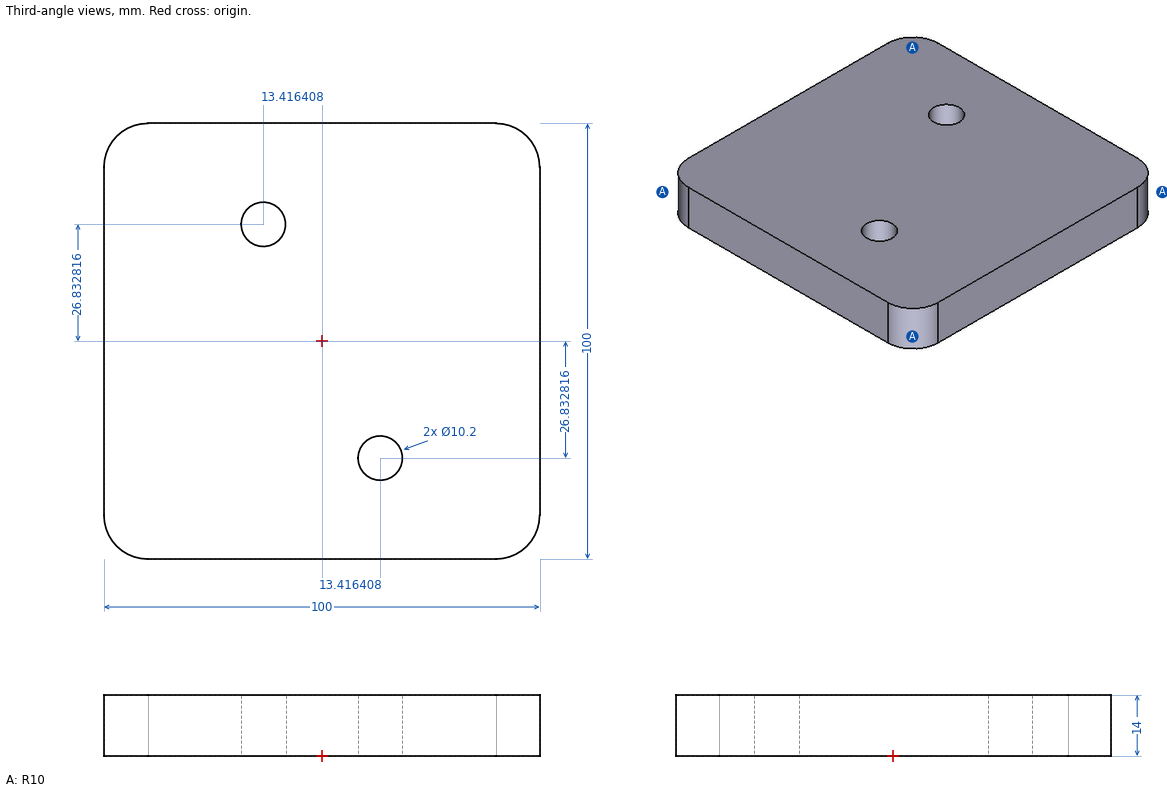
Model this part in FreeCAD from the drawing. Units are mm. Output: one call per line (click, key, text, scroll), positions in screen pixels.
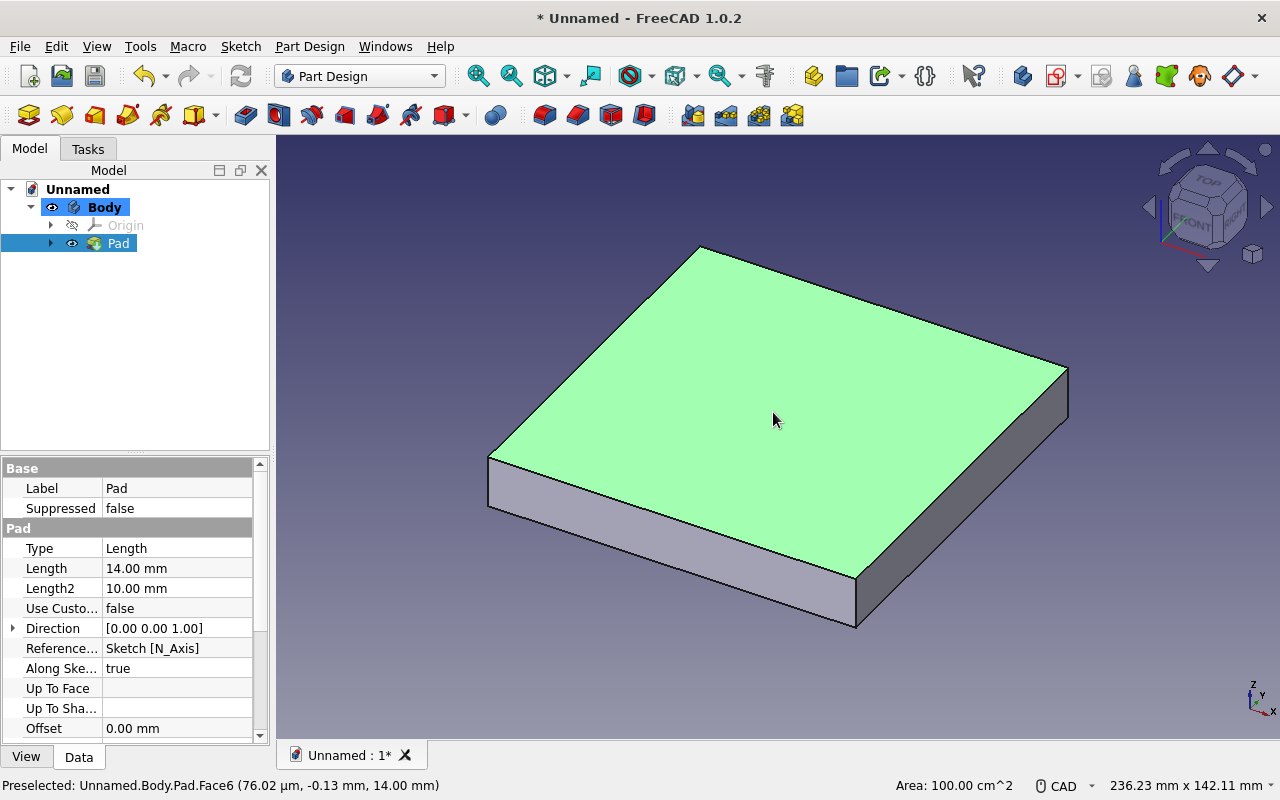
click(1056, 76)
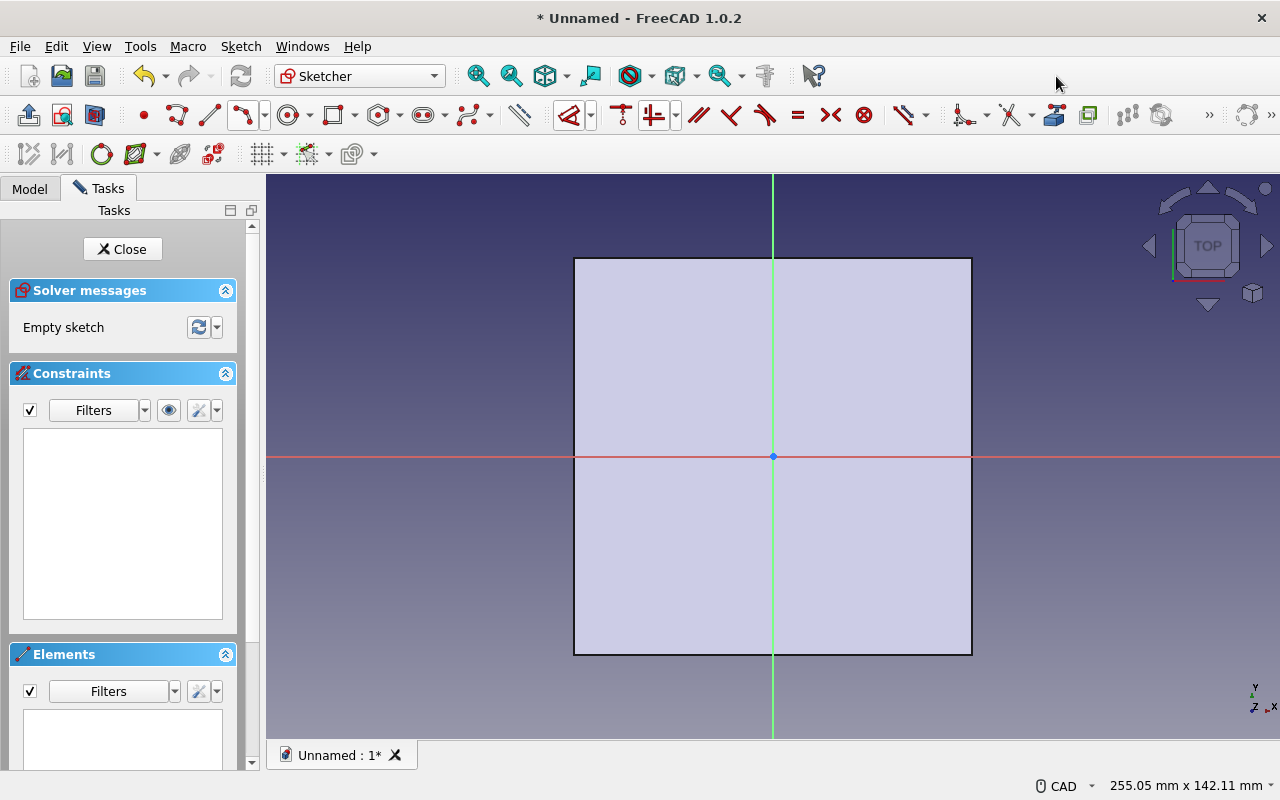
scroll(912, 456, up, 2)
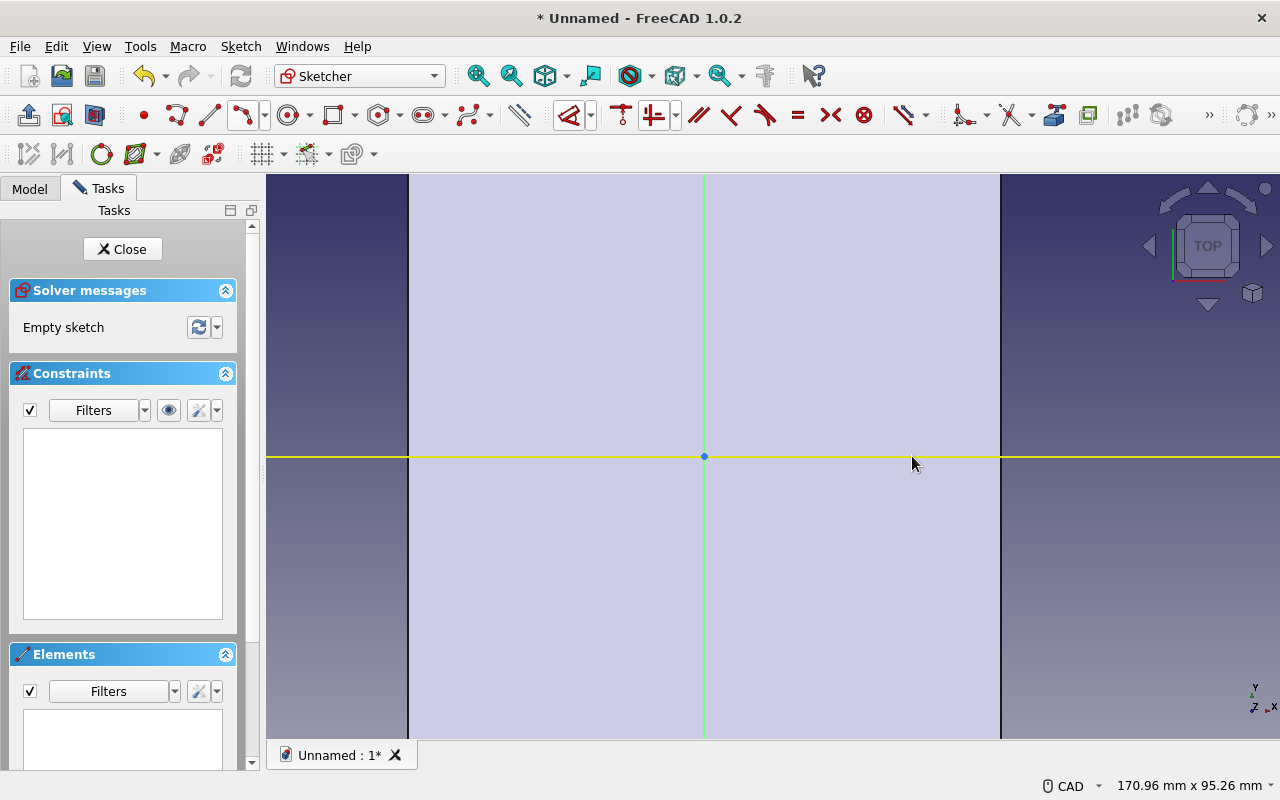
click(288, 116)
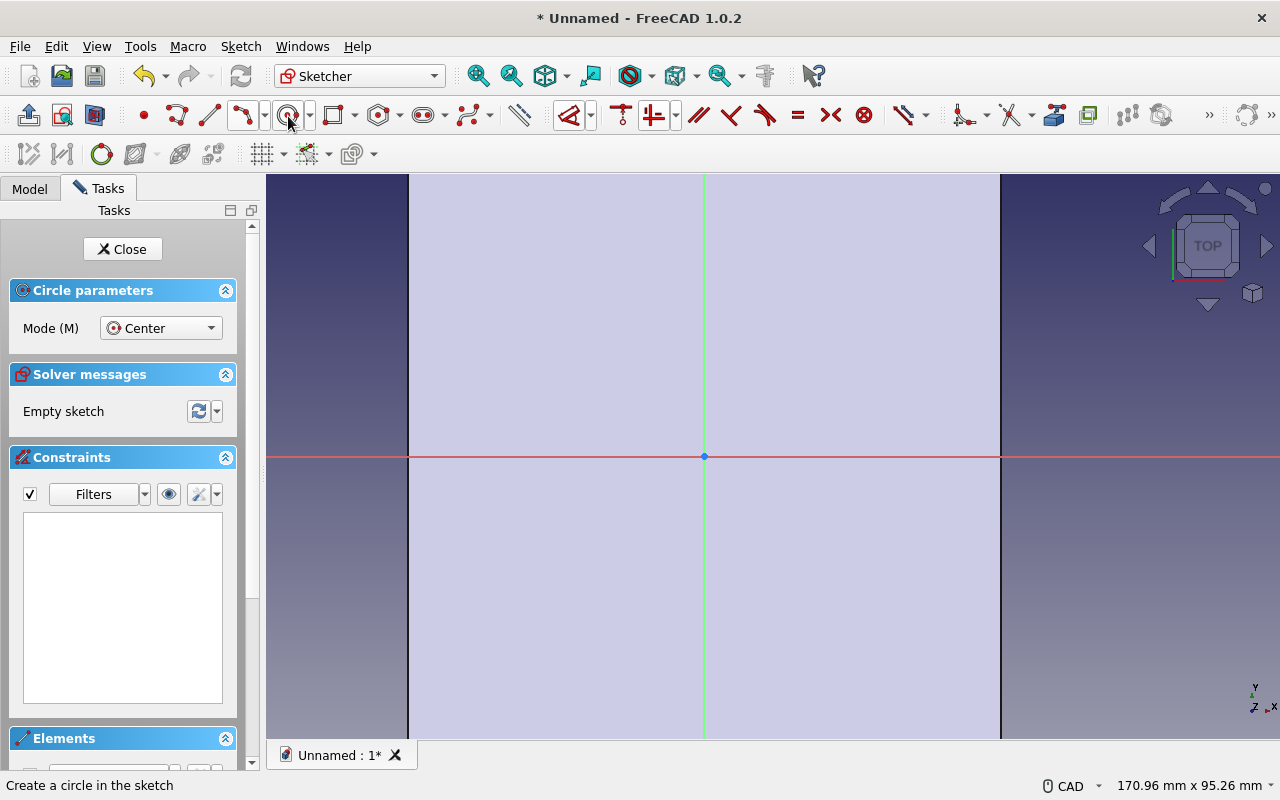
click(784, 616)
click(805, 594)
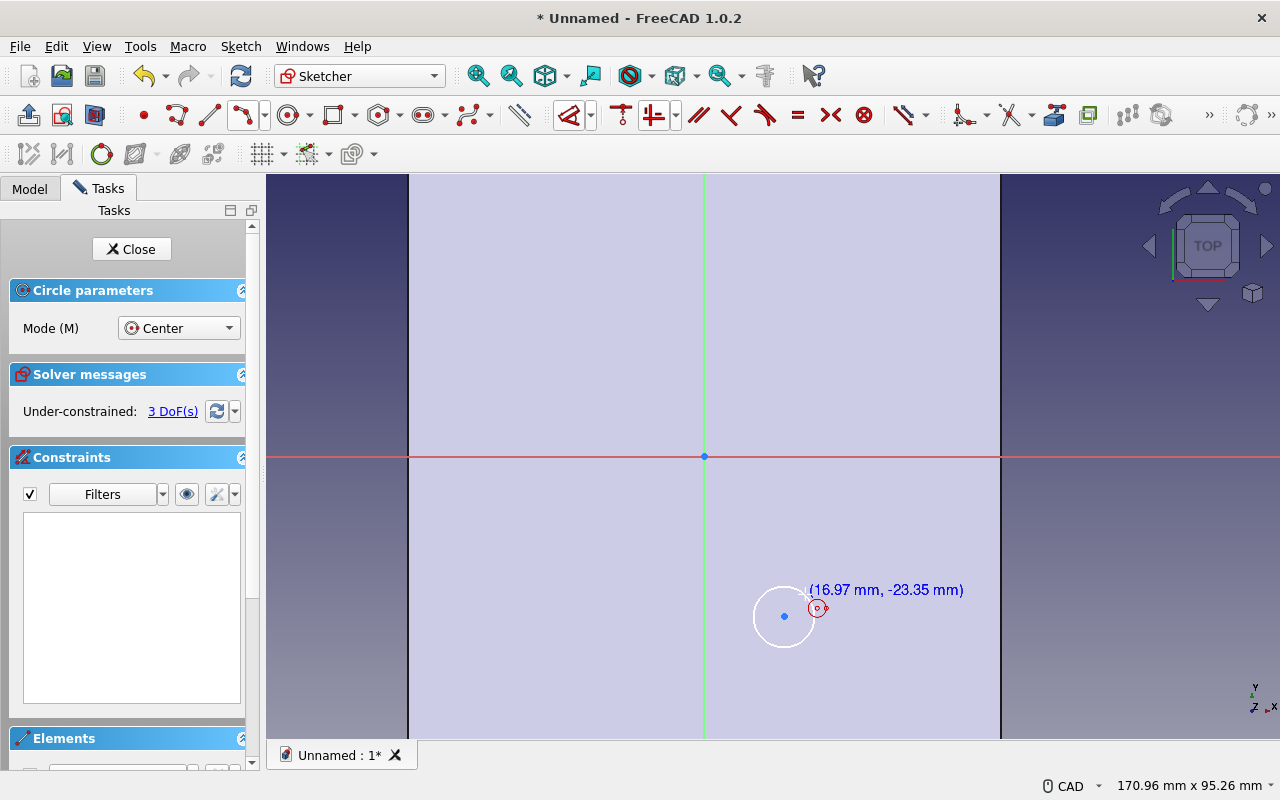
click(625, 297)
click(646, 276)
key(Escape)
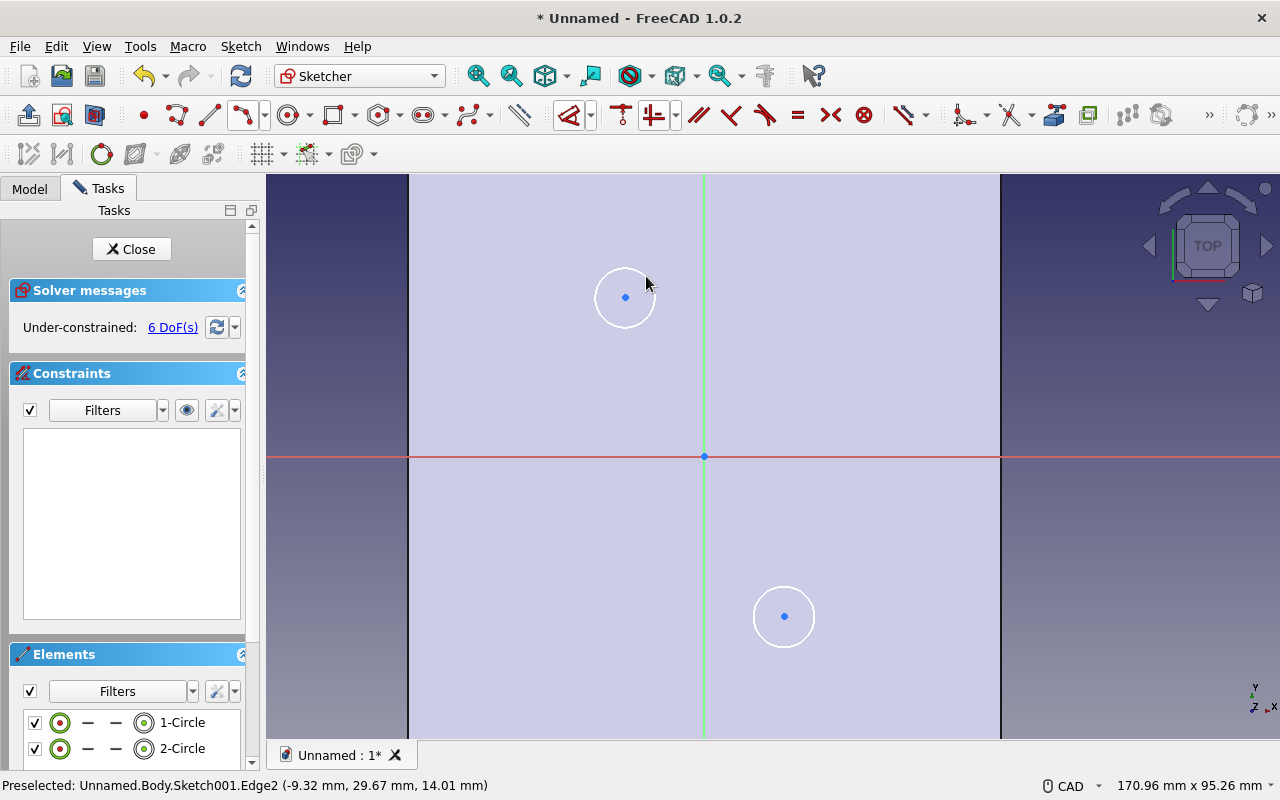
click(805, 595)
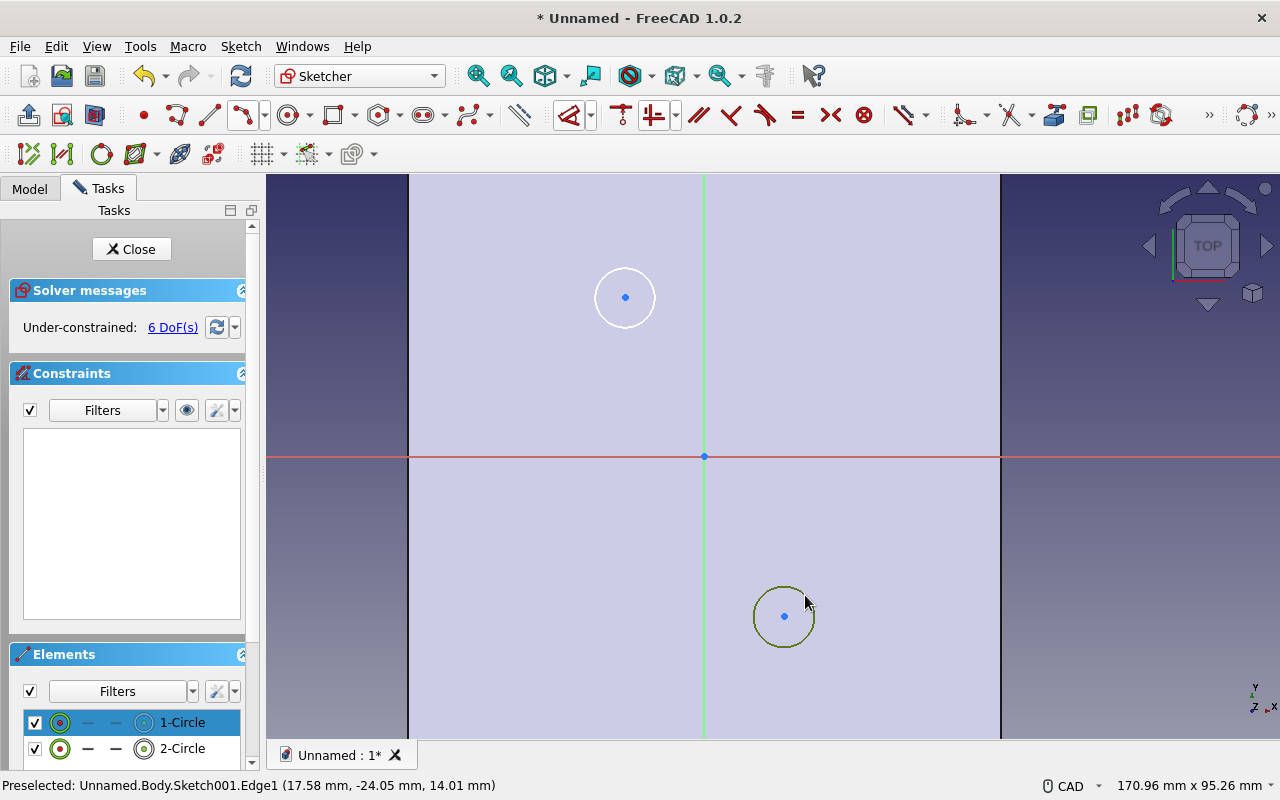
click(646, 277)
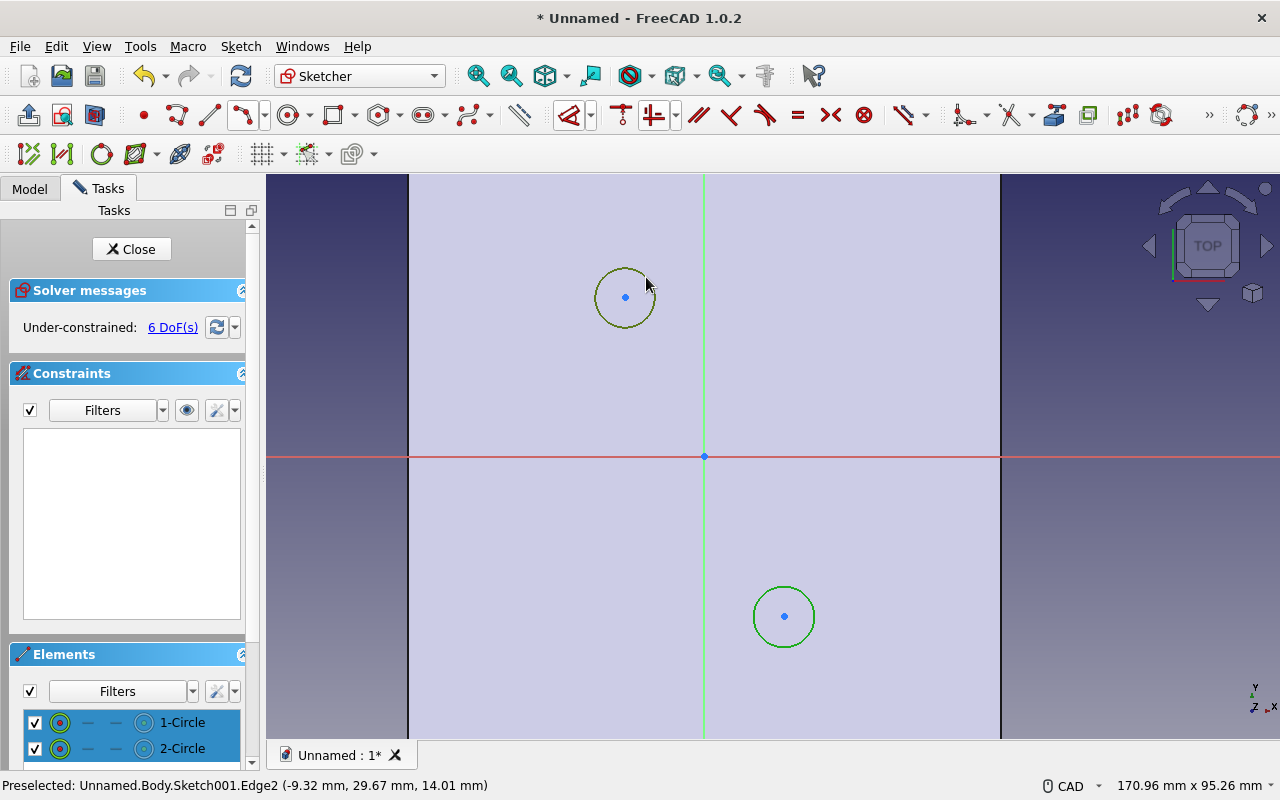
key(e)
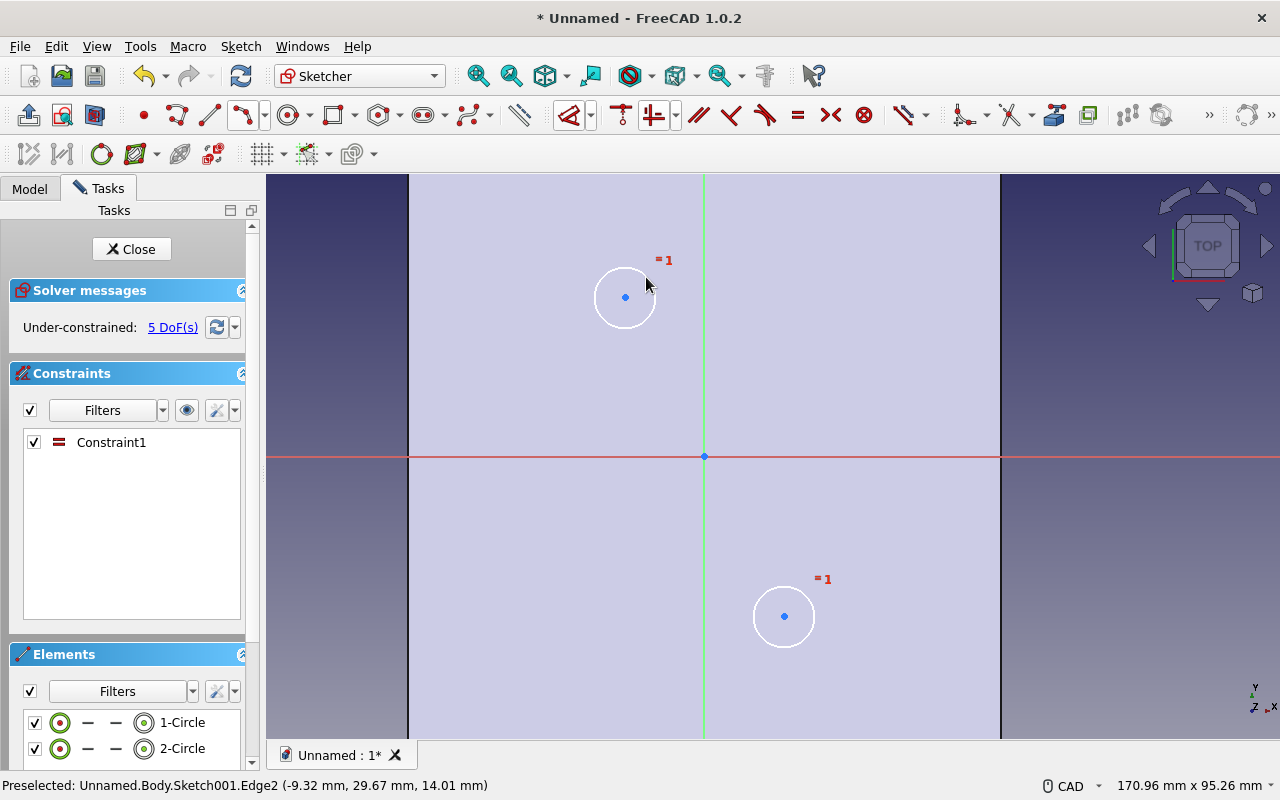
click(805, 595)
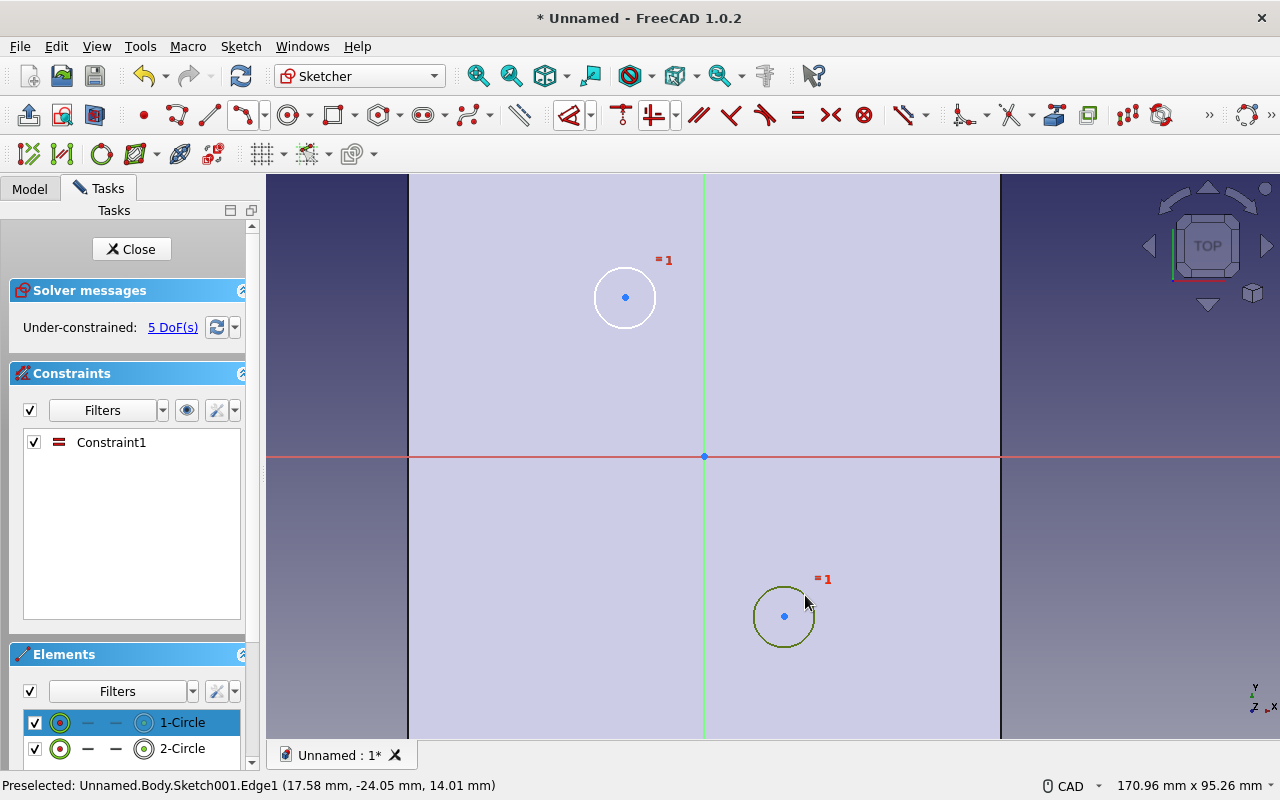
key(k)
key(o)